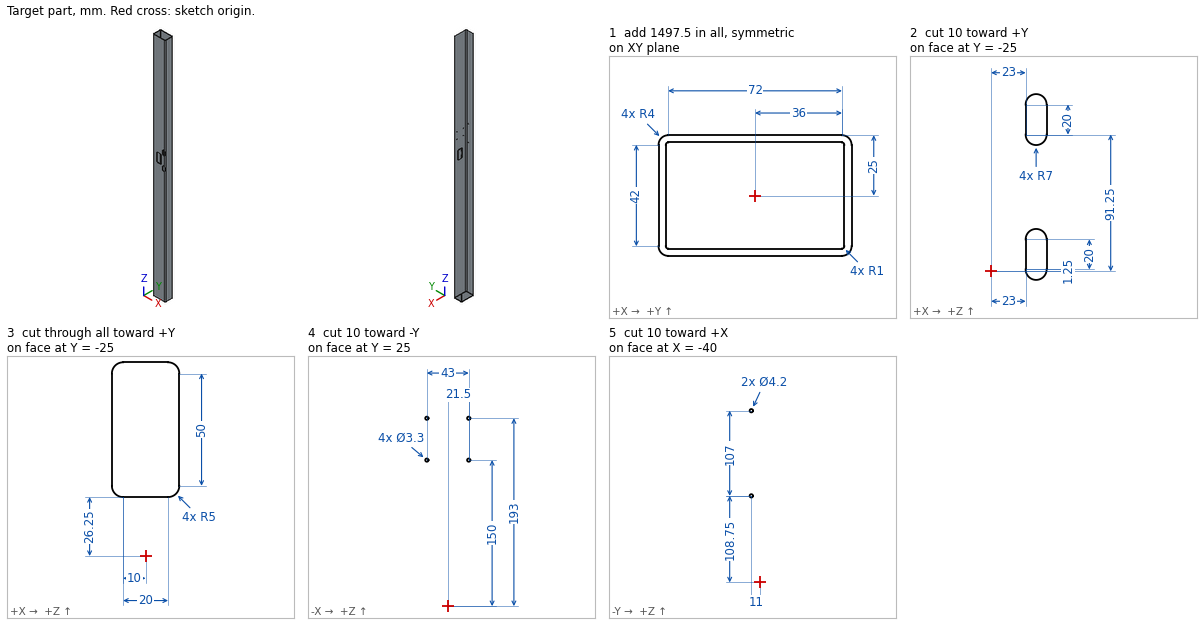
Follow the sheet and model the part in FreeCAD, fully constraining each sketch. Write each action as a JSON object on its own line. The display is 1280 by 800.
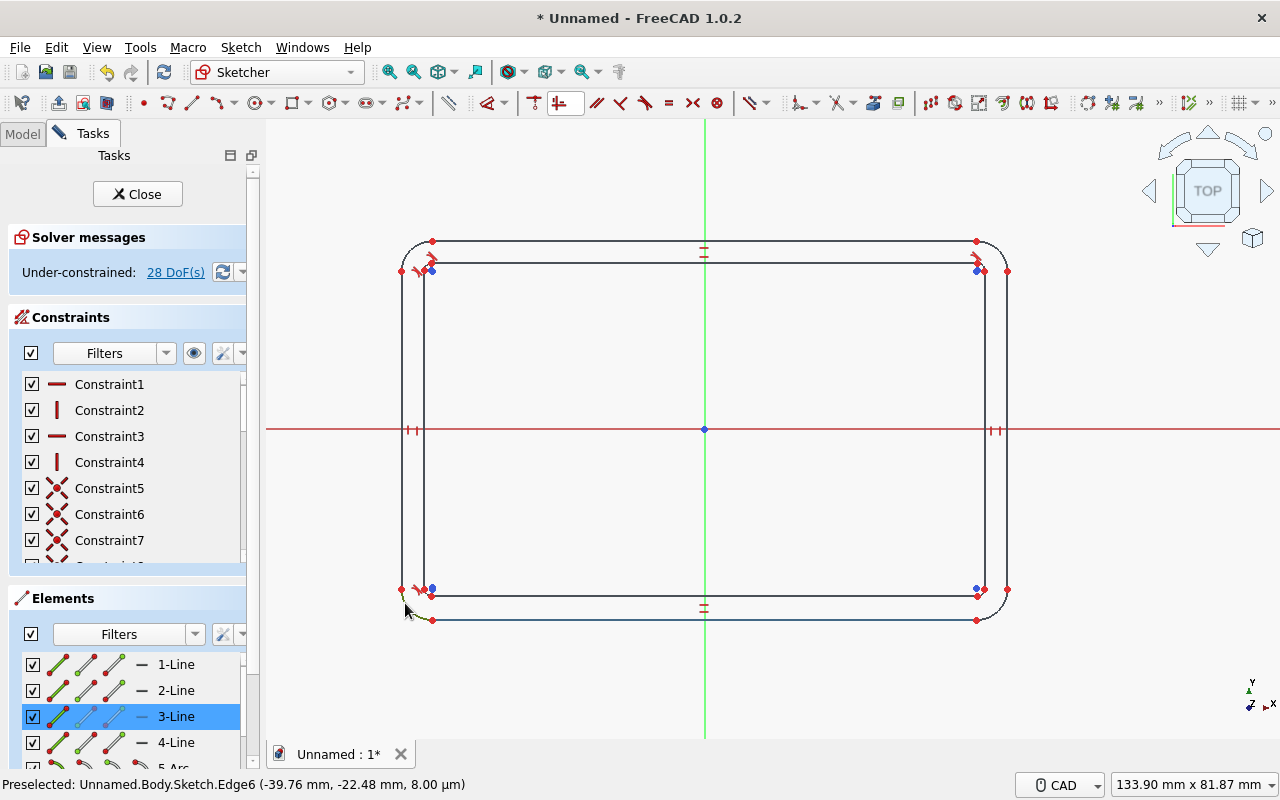
{"action": "key", "text": "t"}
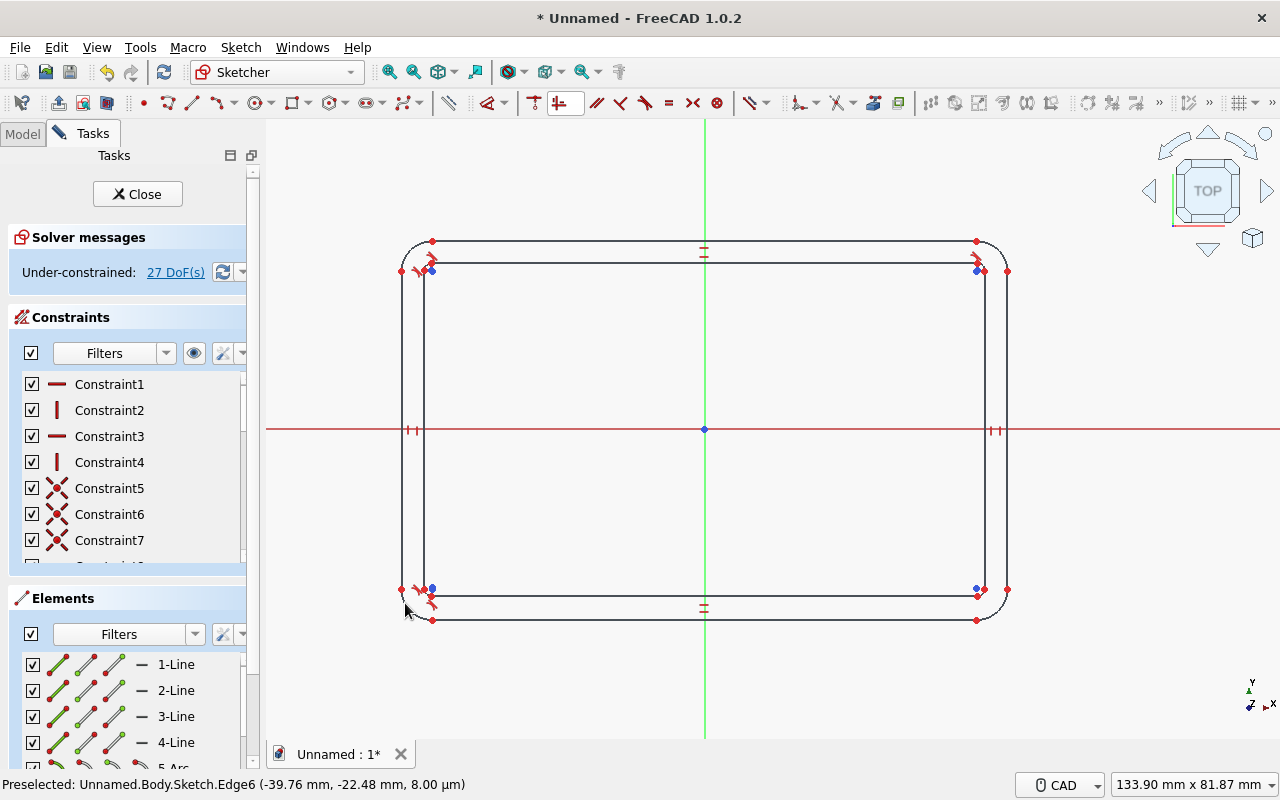
{"action": "left_click", "coordinate": [596, 620]}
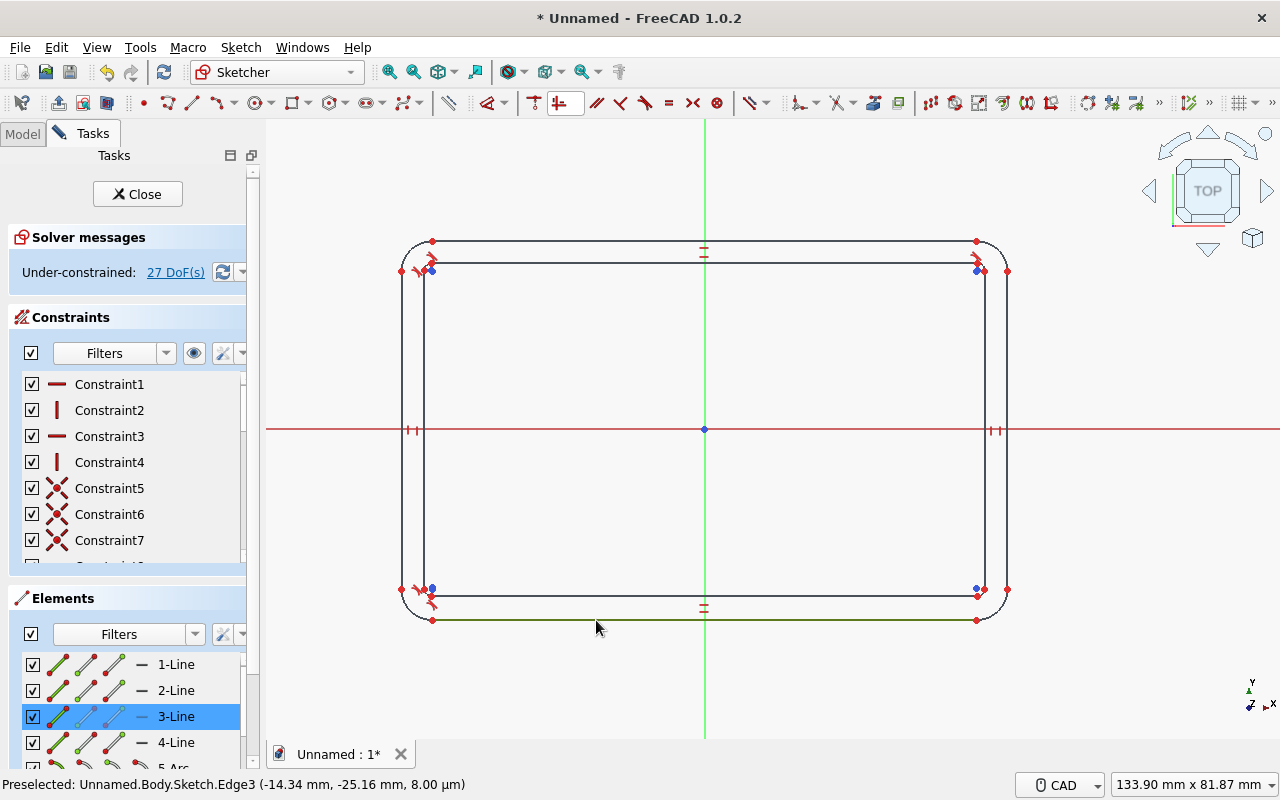
{"action": "left_click", "coordinate": [991, 616]}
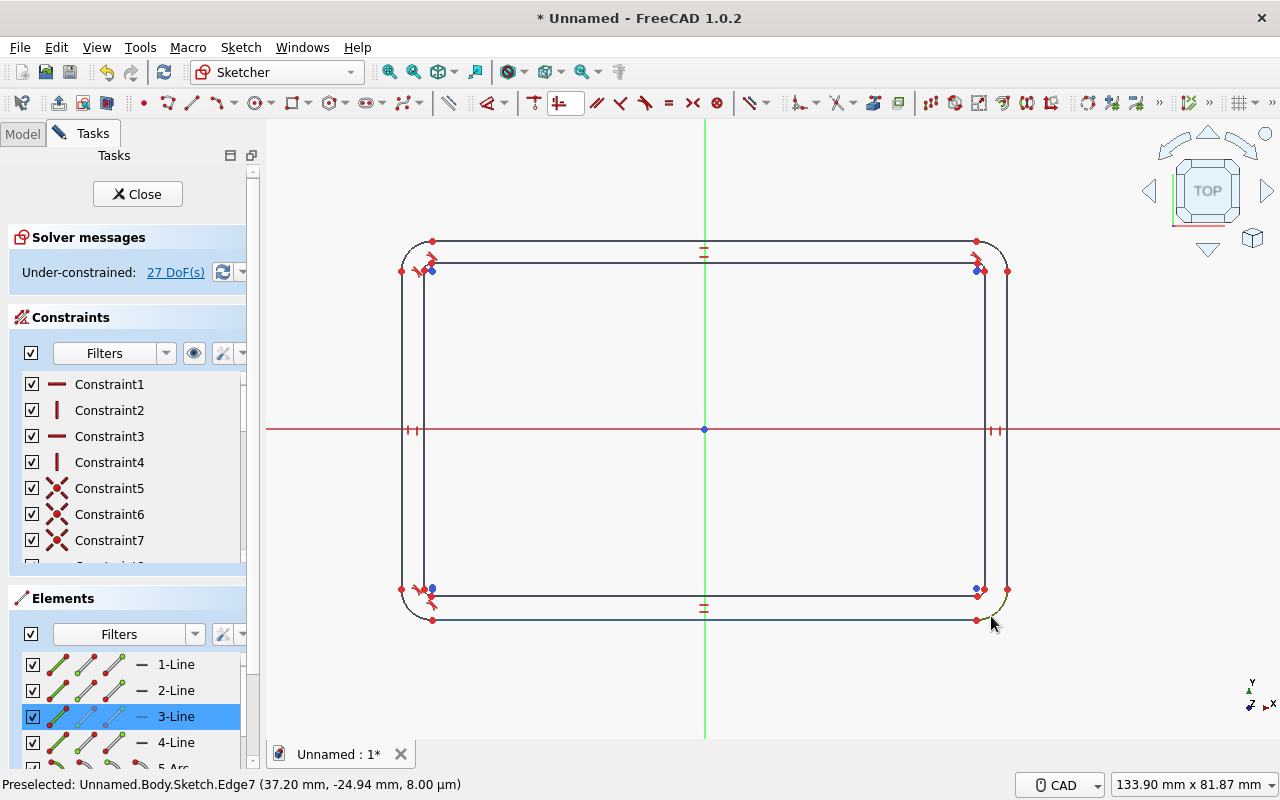
{"action": "key", "text": "t"}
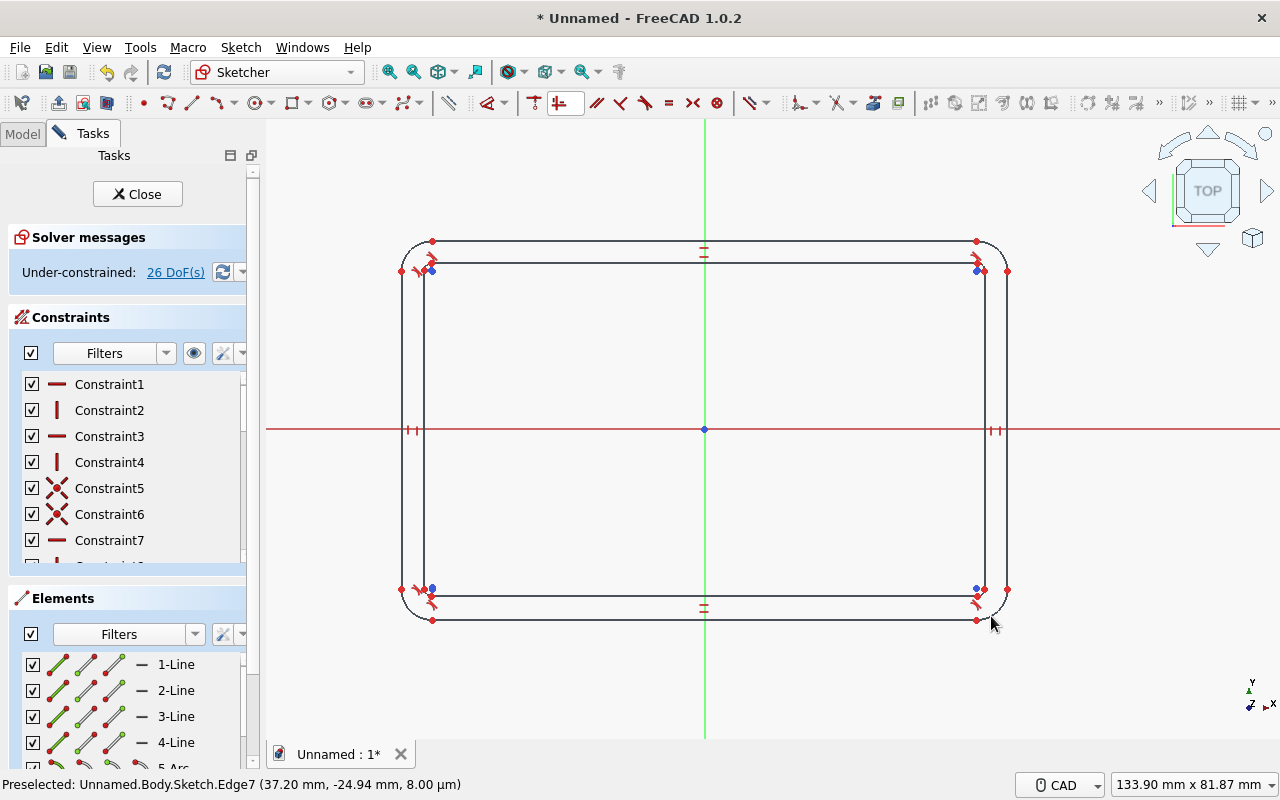
{"action": "left_click", "coordinate": [1007, 494]}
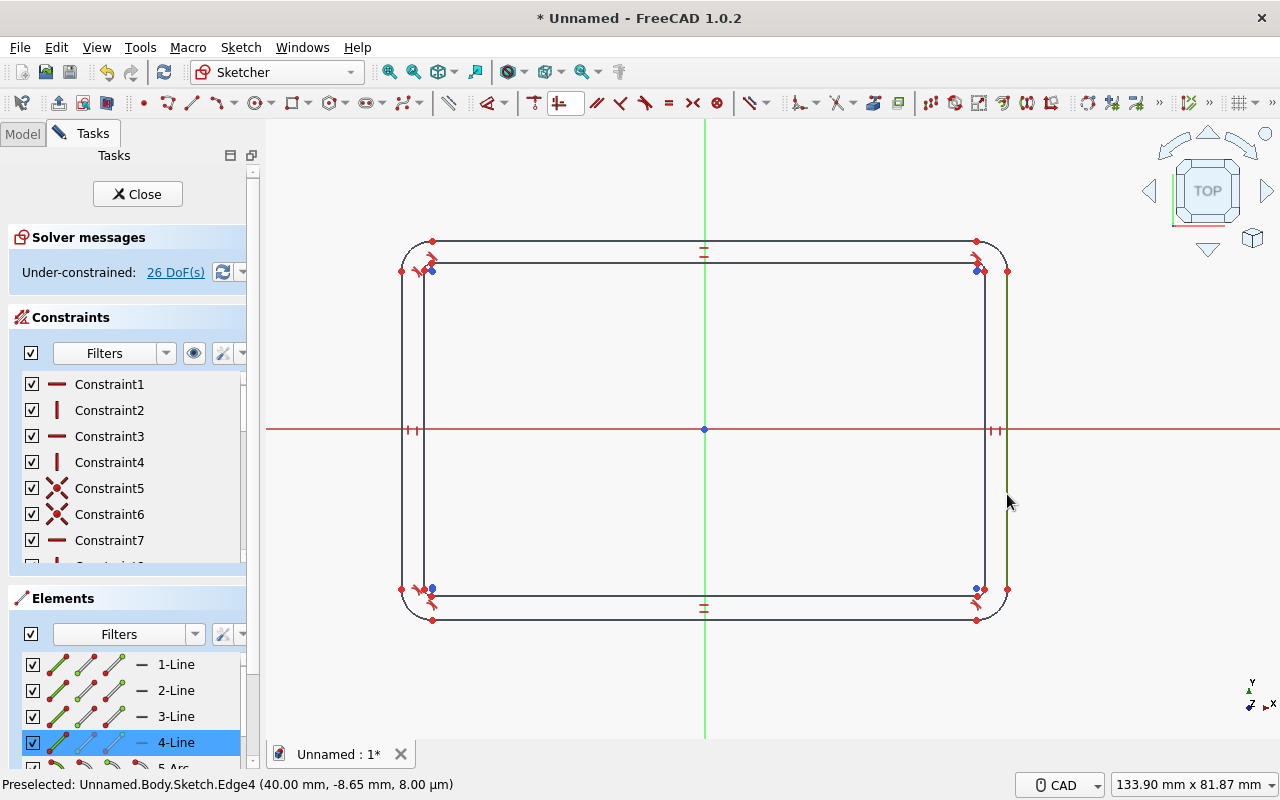
{"action": "left_click", "coordinate": [990, 617]}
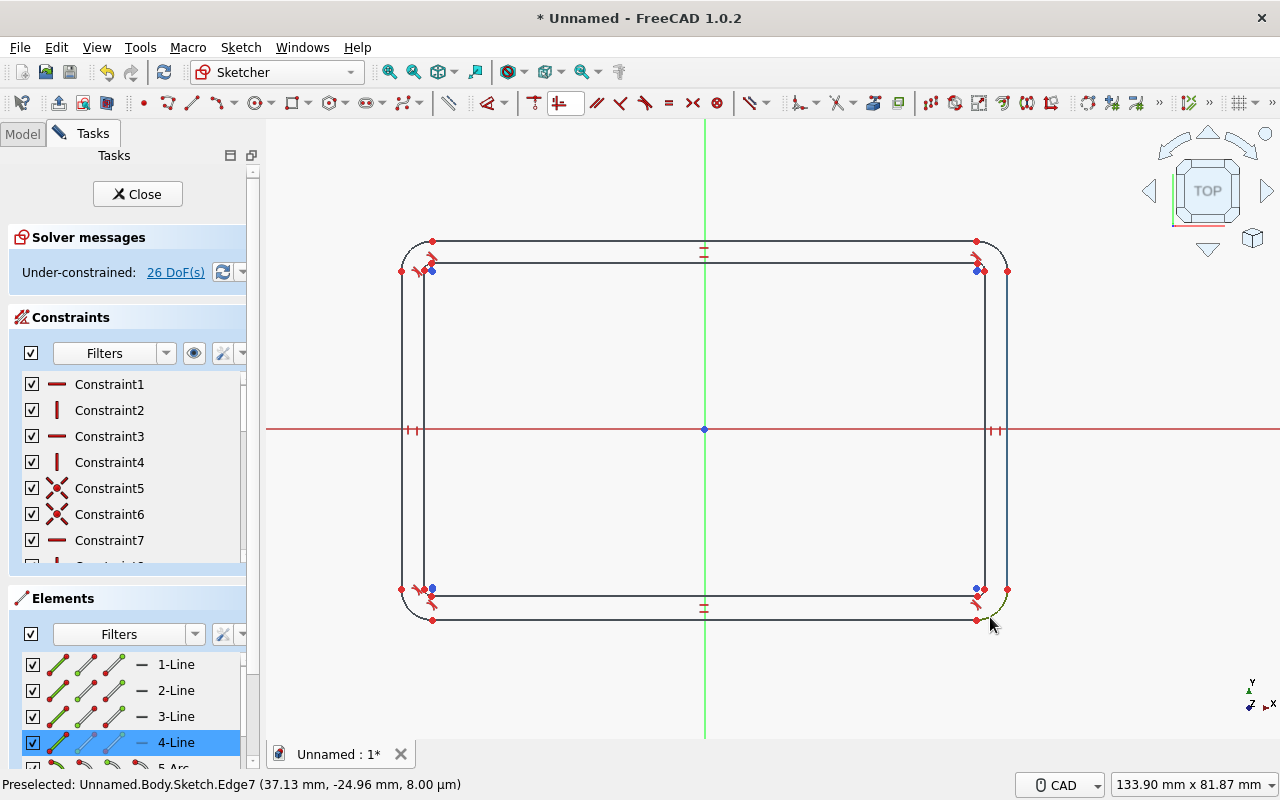
{"action": "left_click", "coordinate": [646, 104]}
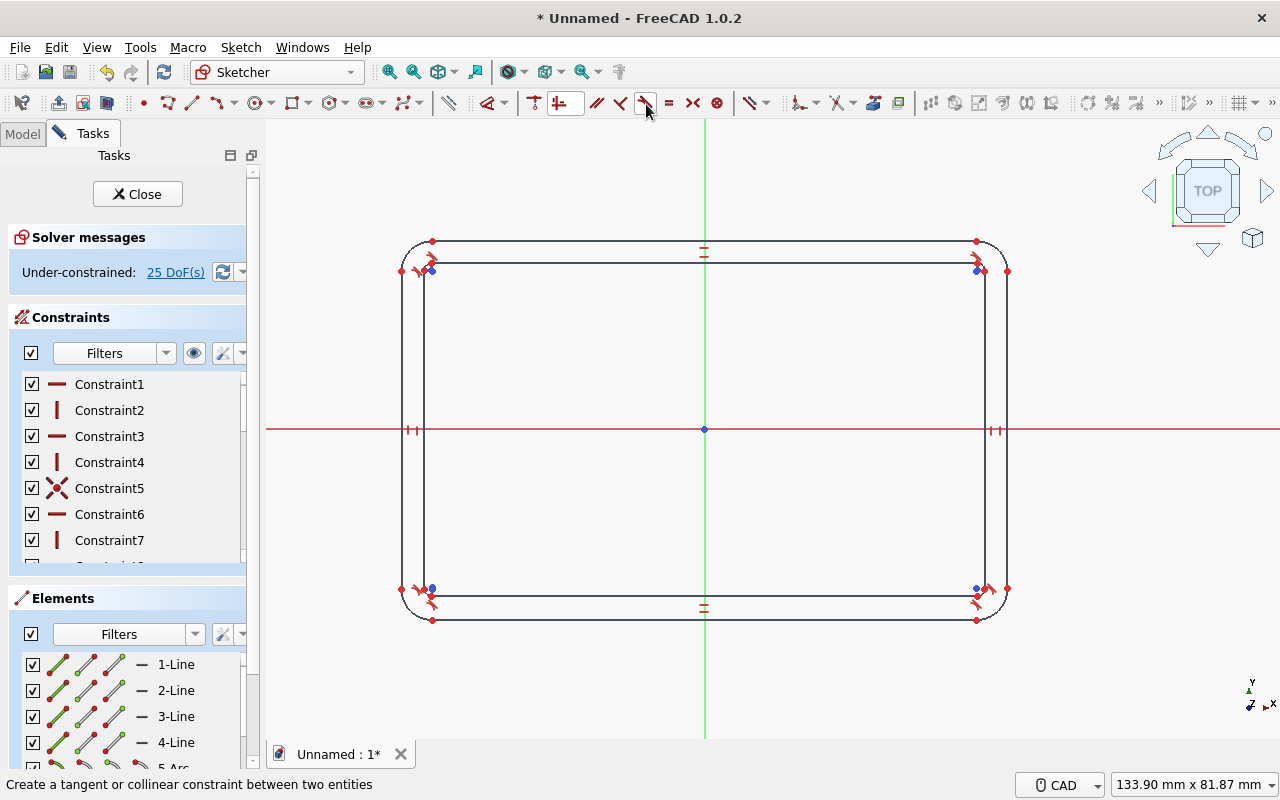
{"action": "left_click", "coordinate": [1007, 494]}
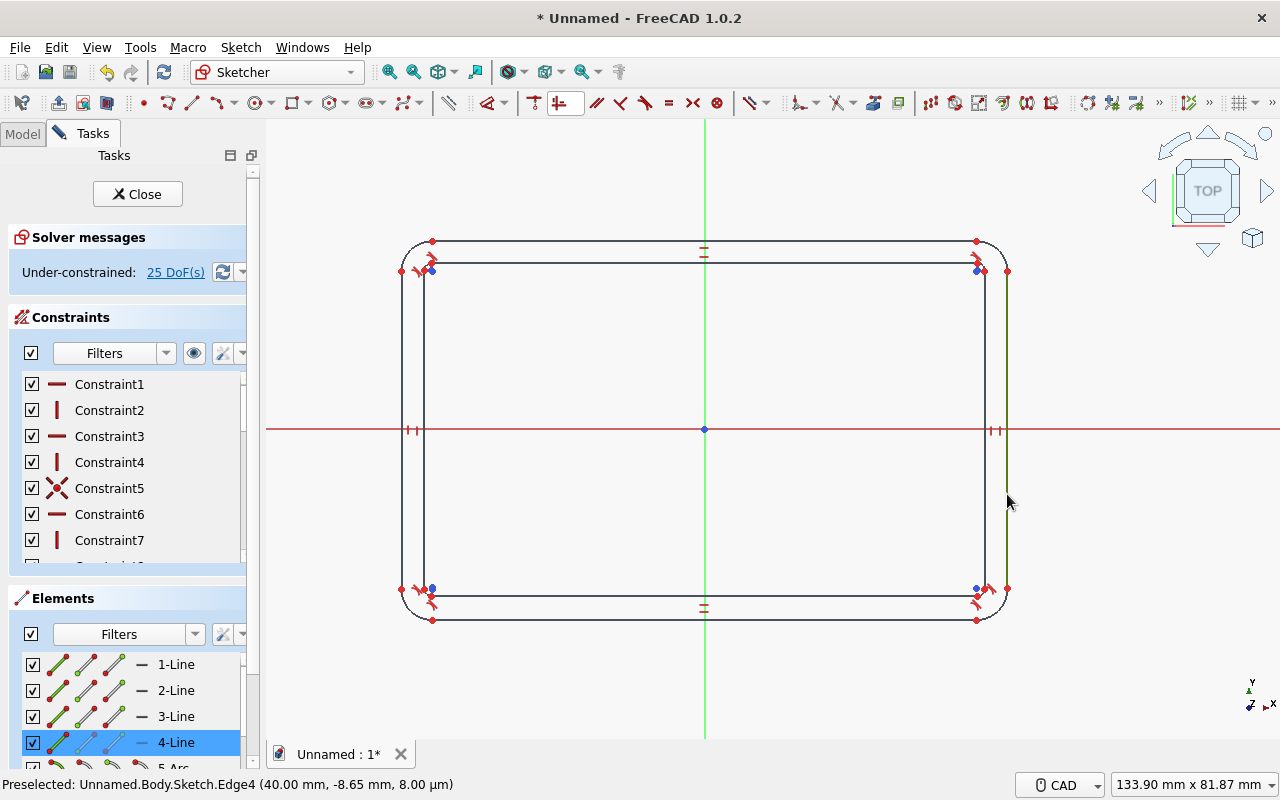
{"action": "left_click", "coordinate": [1004, 258]}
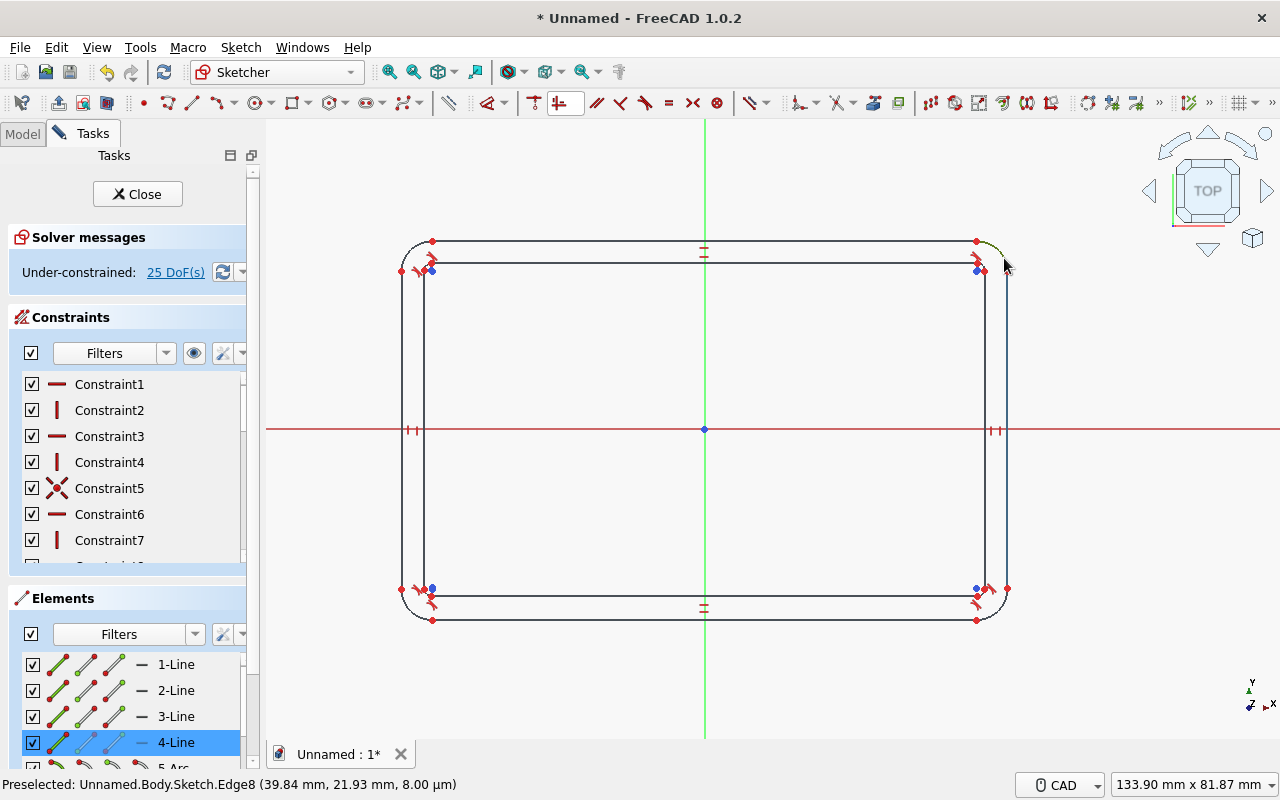
{"action": "key", "text": "t"}